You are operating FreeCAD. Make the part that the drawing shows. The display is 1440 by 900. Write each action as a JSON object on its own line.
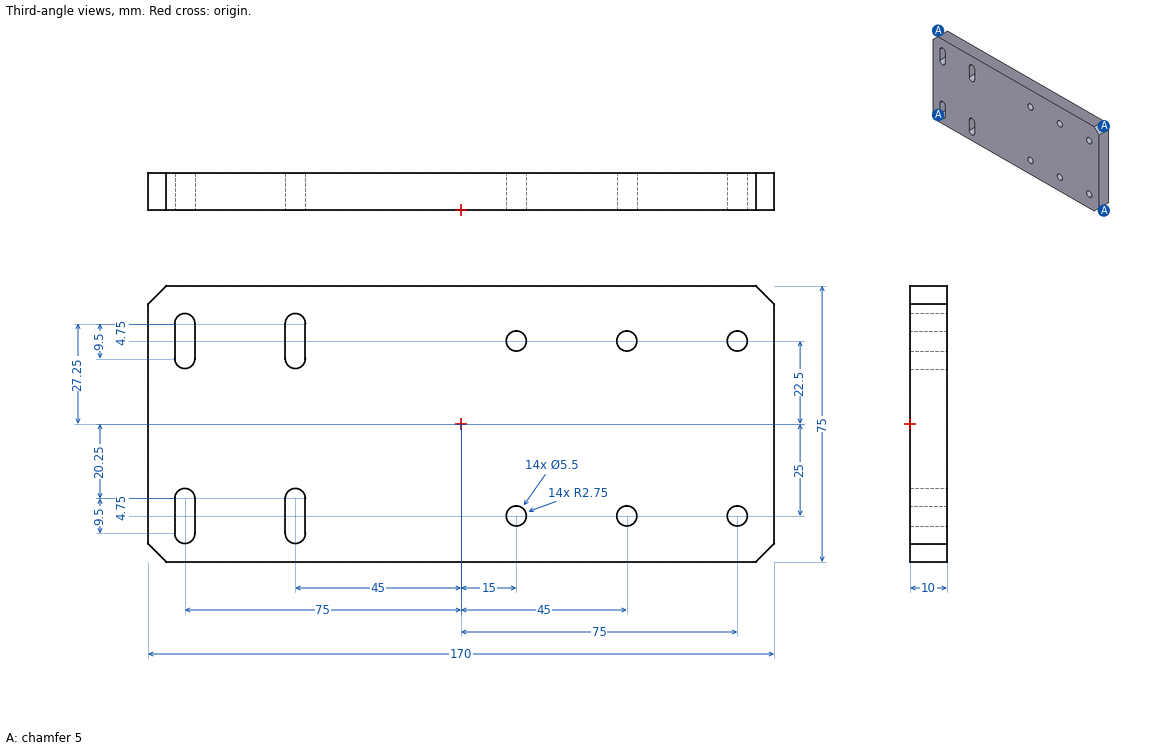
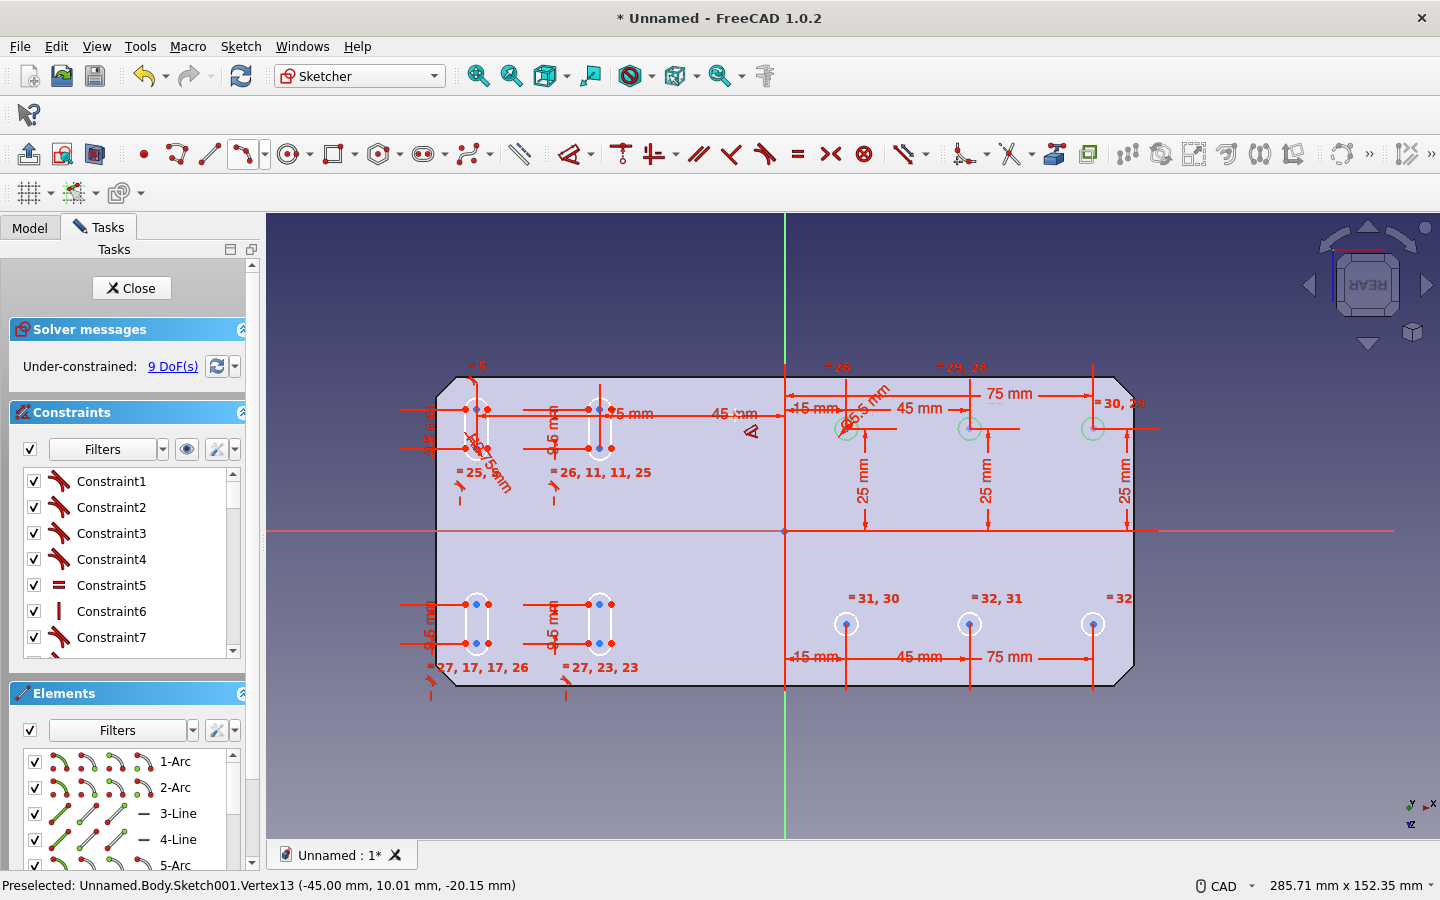
{"action": "left_click", "coordinate": [477, 644]}
{"action": "left_click", "coordinate": [631, 678]}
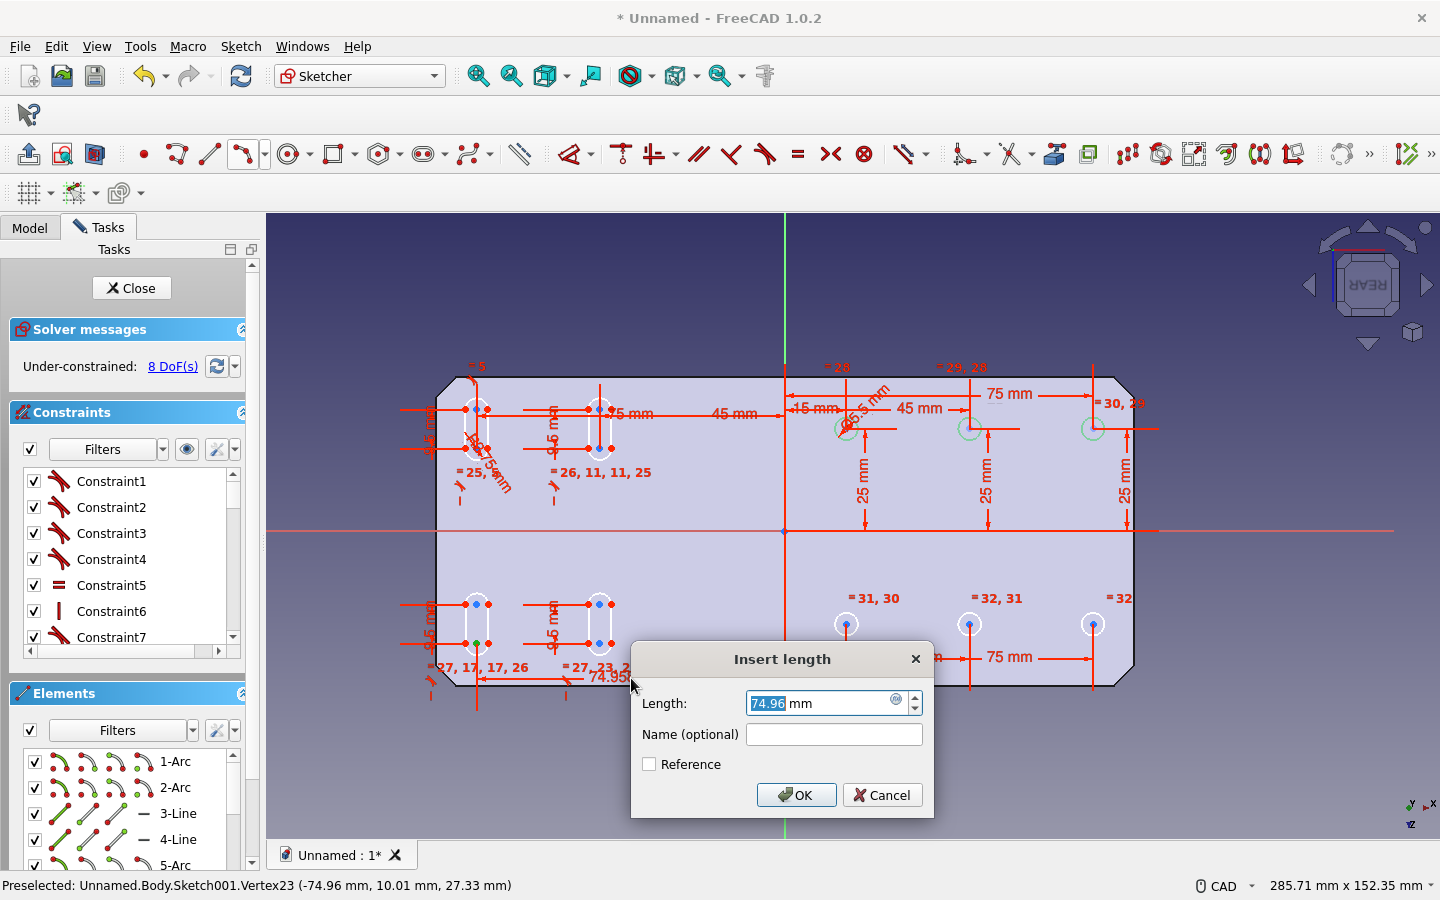
{"action": "type", "text": "75"}
{"action": "key", "text": "Return"}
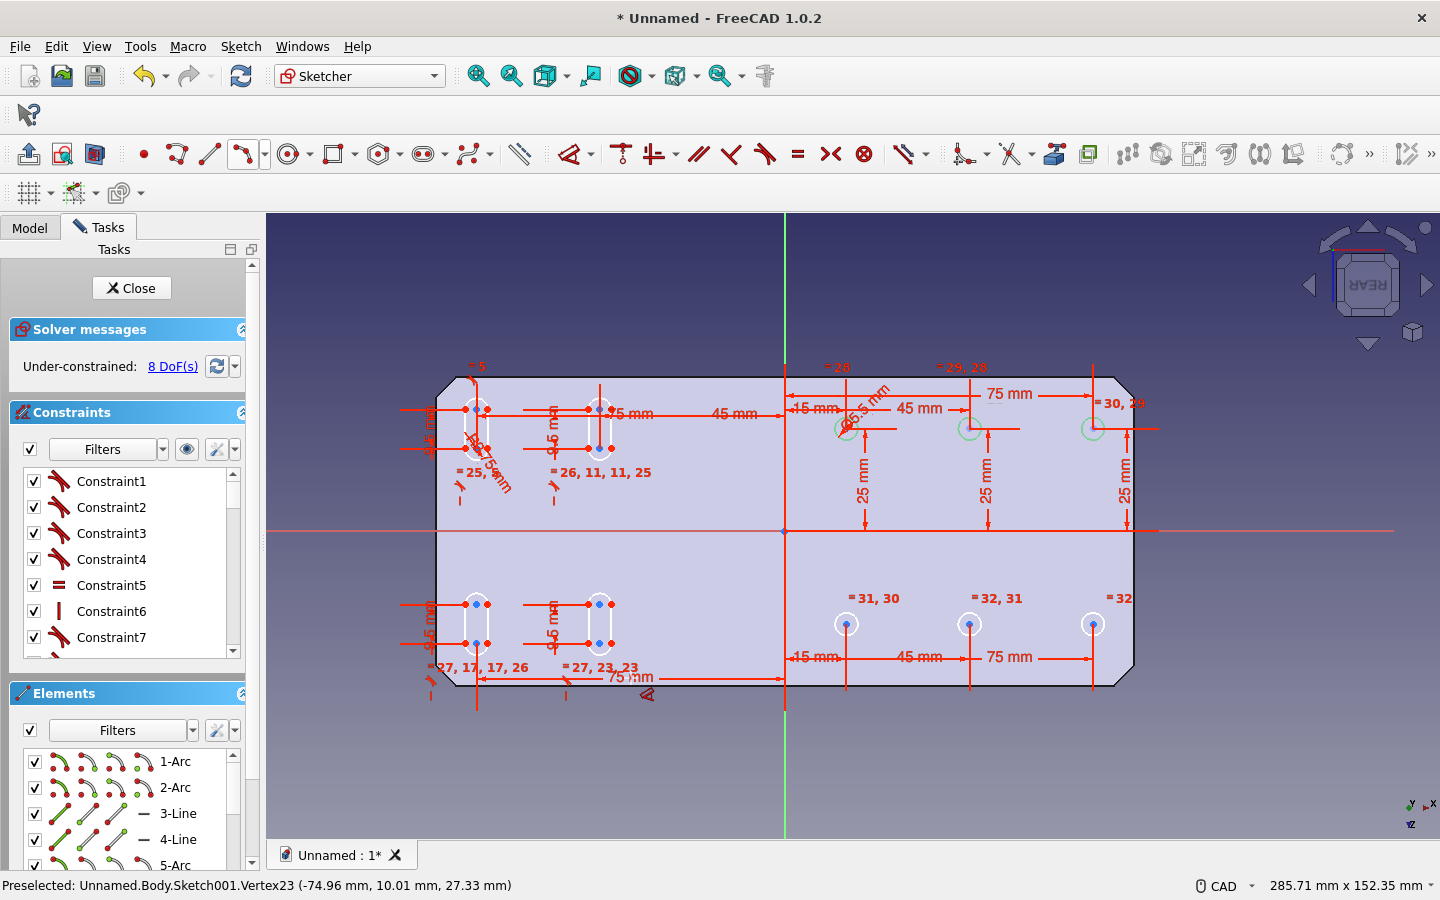
{"action": "left_click", "coordinate": [600, 644]}
{"action": "left_click", "coordinate": [735, 678]}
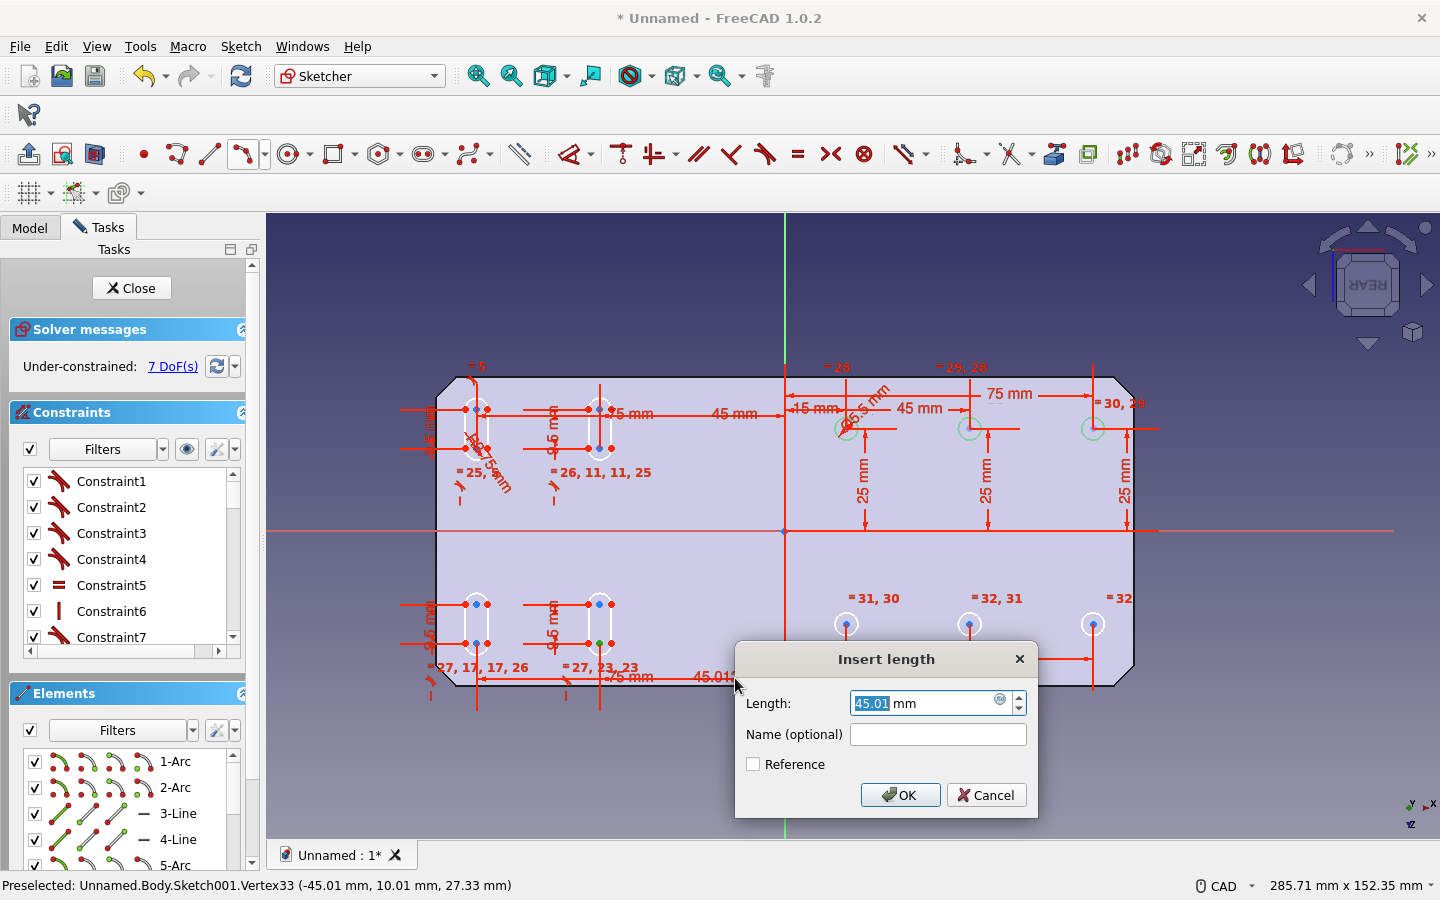
{"action": "type", "text": "45"}
{"action": "key", "text": "Return"}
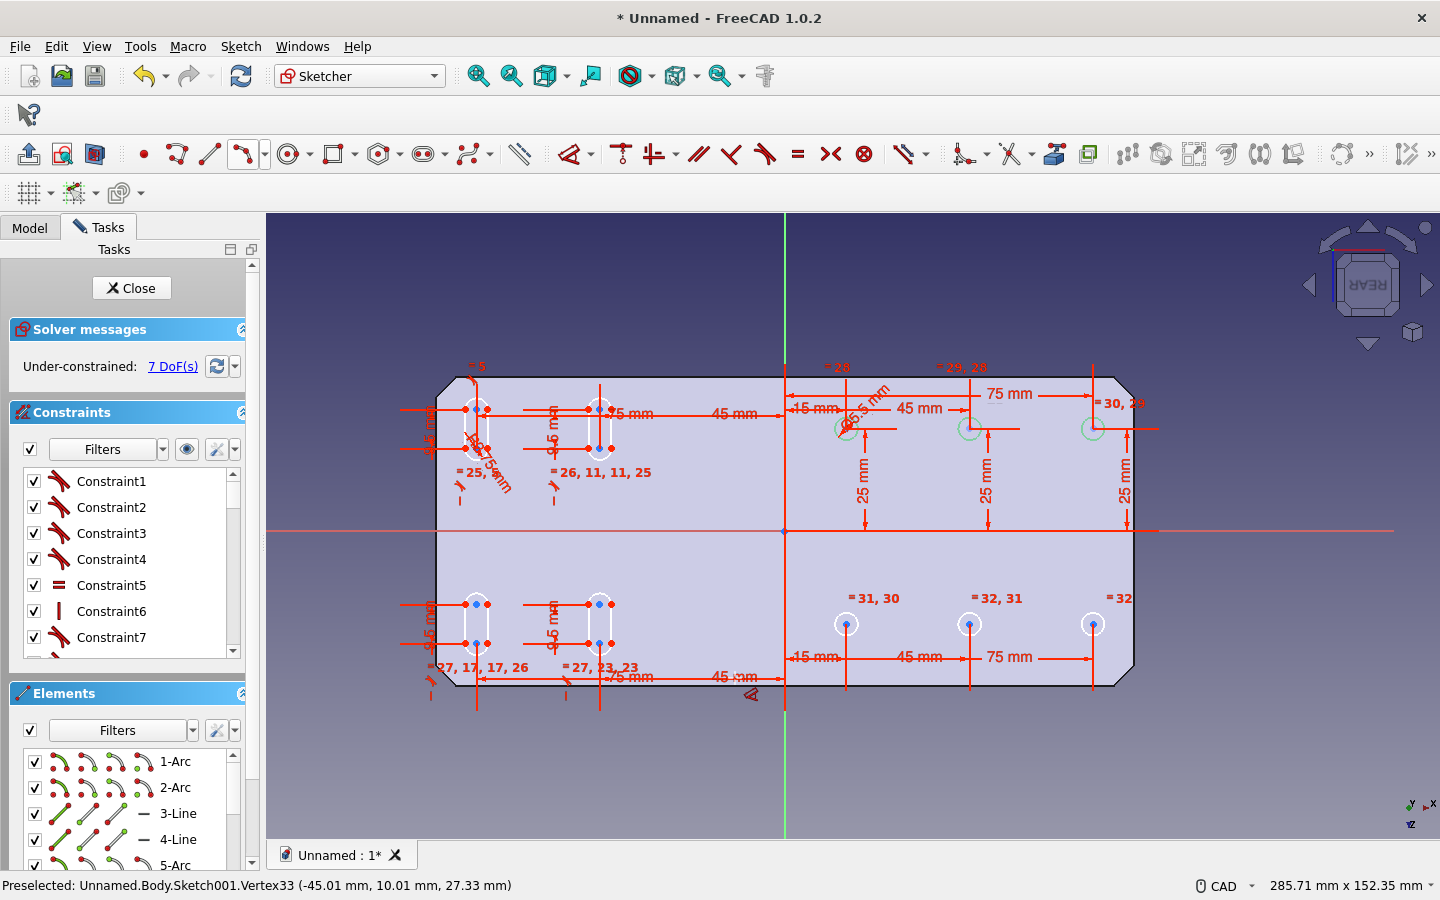
{"action": "left_click", "coordinate": [846, 624]}
{"action": "left_click", "coordinate": [880, 578]}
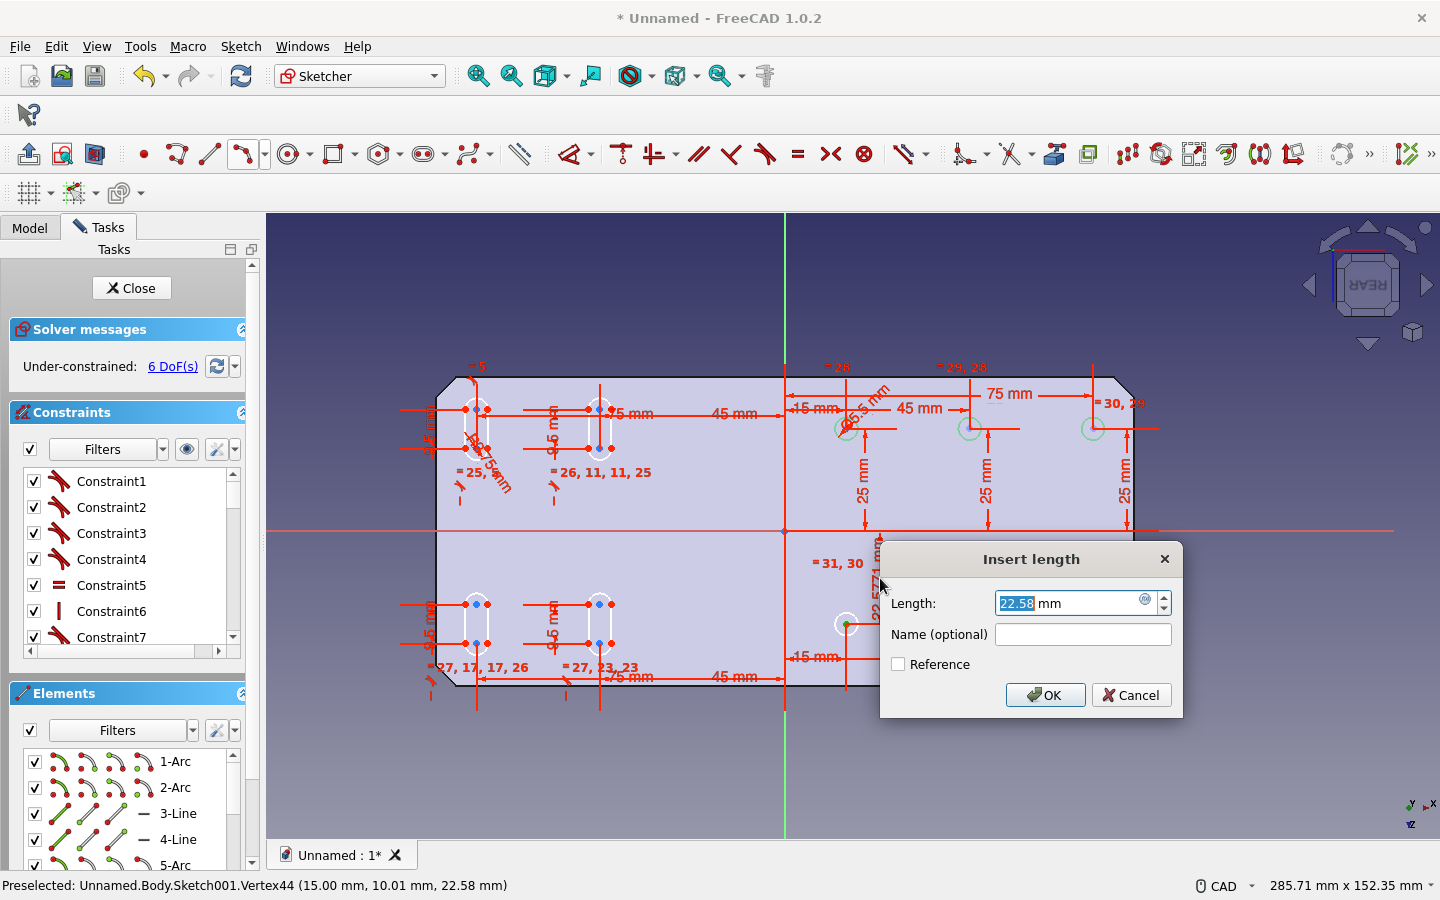
{"action": "type", "text": "22.5"}
{"action": "key", "text": "Return"}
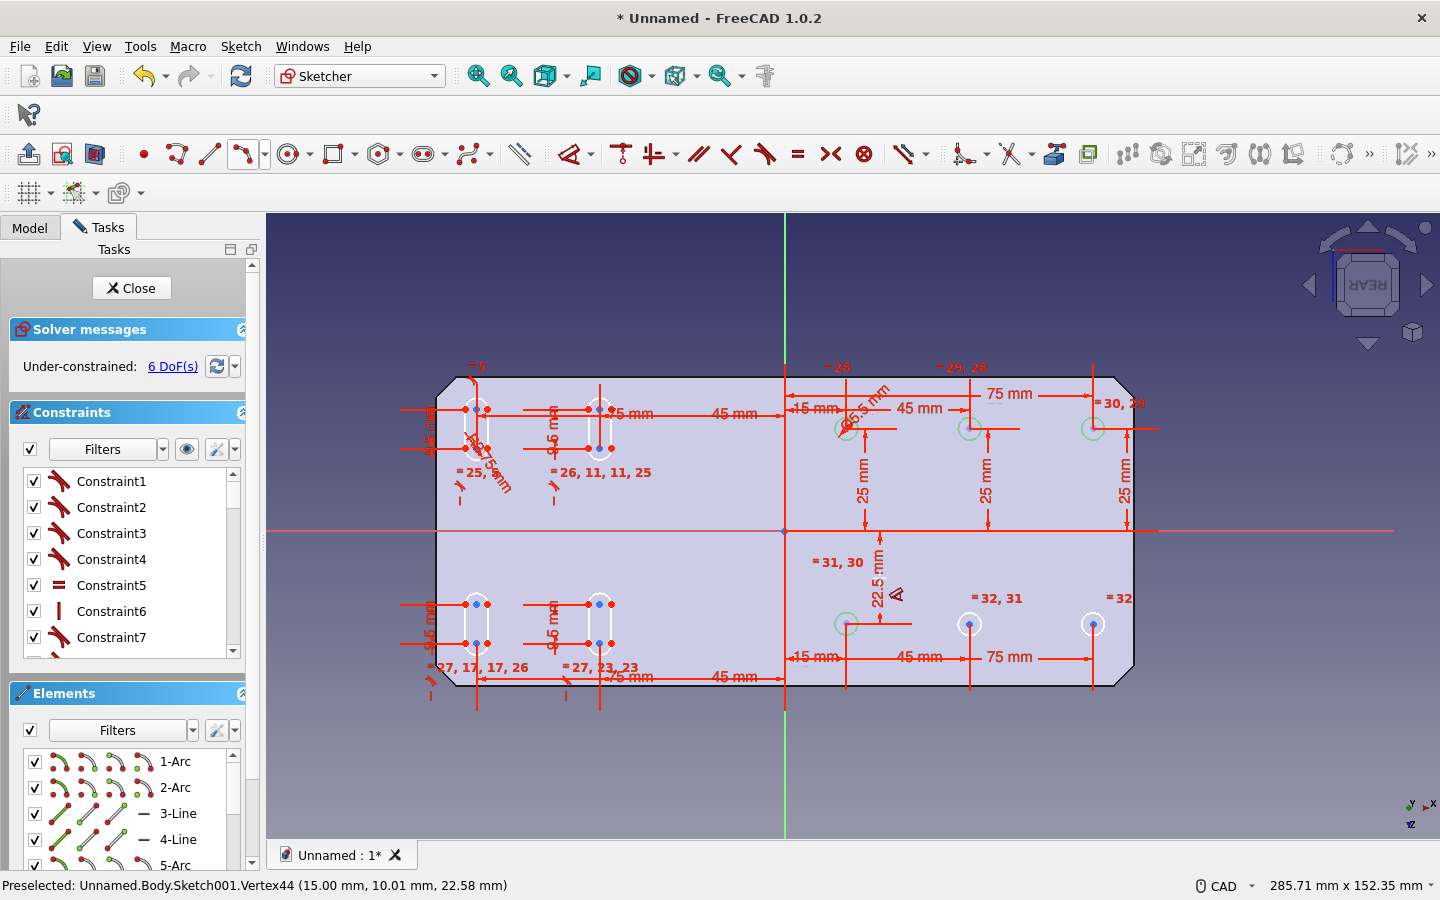
{"action": "left_click", "coordinate": [970, 624]}
{"action": "left_click", "coordinate": [1004, 578]}